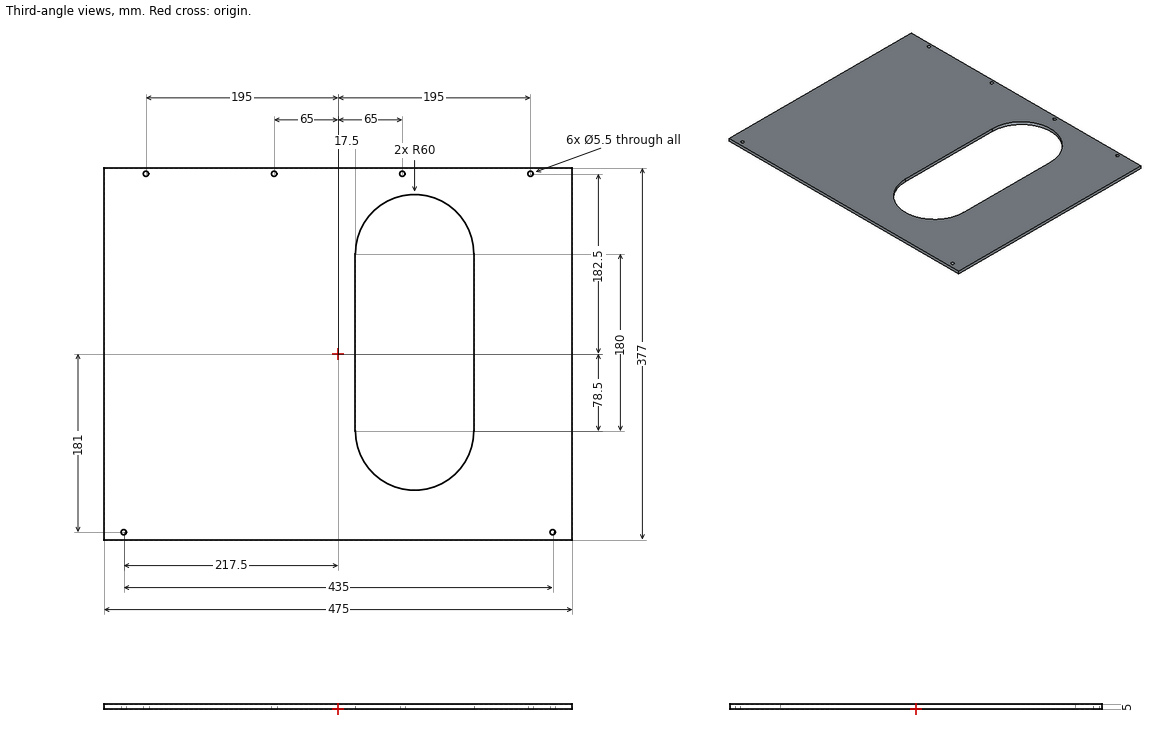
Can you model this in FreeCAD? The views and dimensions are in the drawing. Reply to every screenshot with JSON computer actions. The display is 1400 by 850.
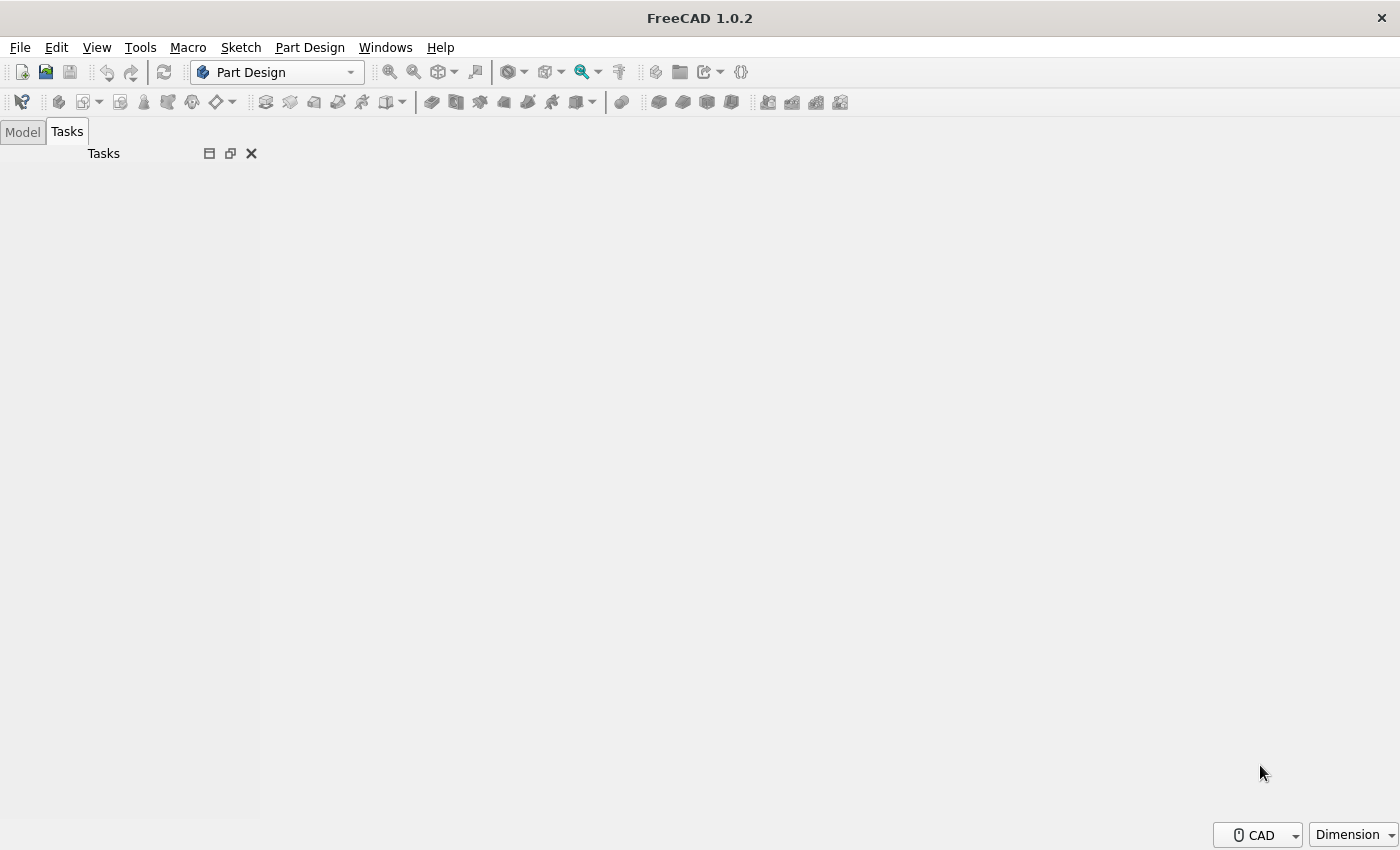
{"action": "key", "text": "ctrl+n"}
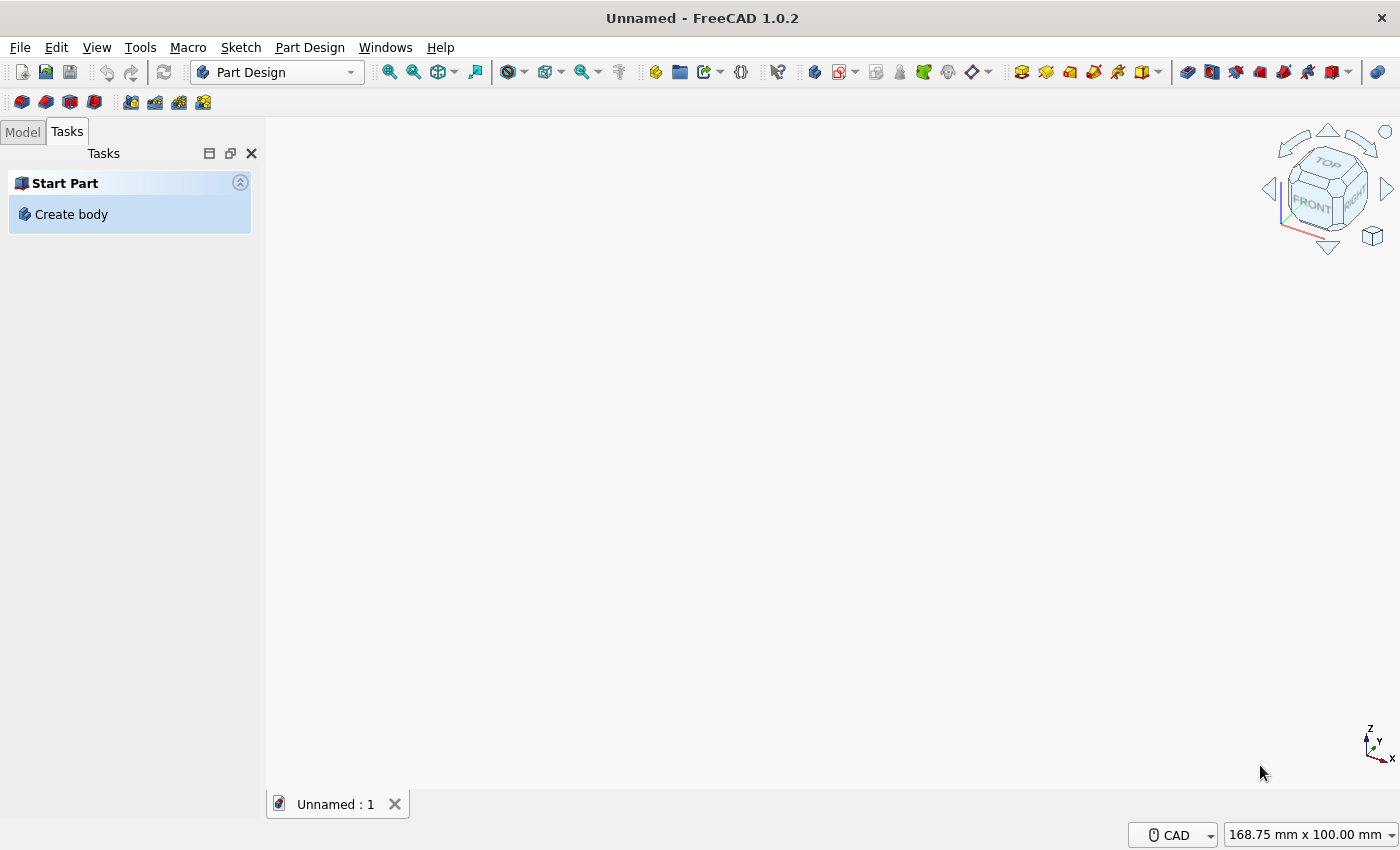
{"action": "left_click", "coordinate": [840, 72]}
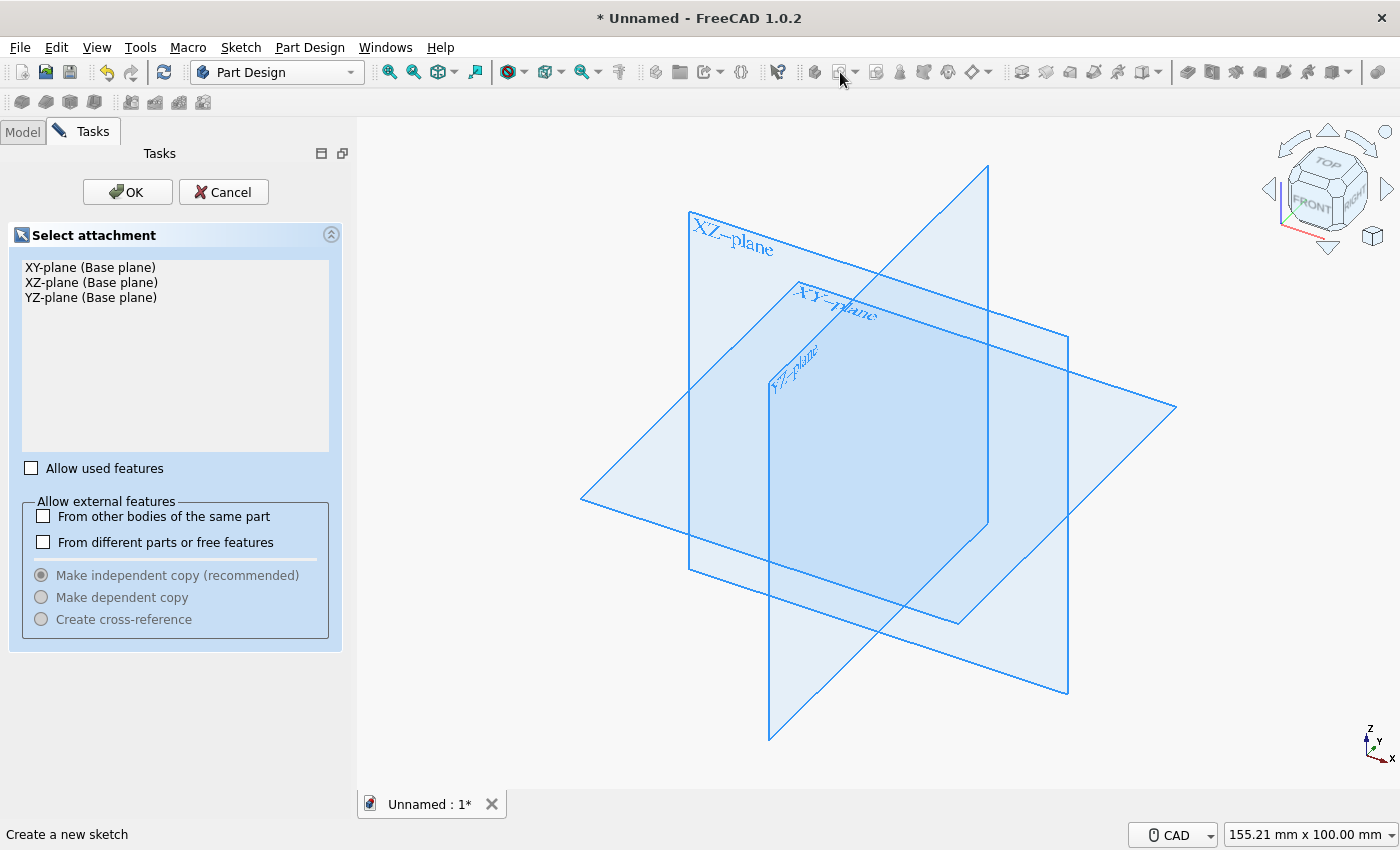
{"action": "left_click", "coordinate": [82, 268]}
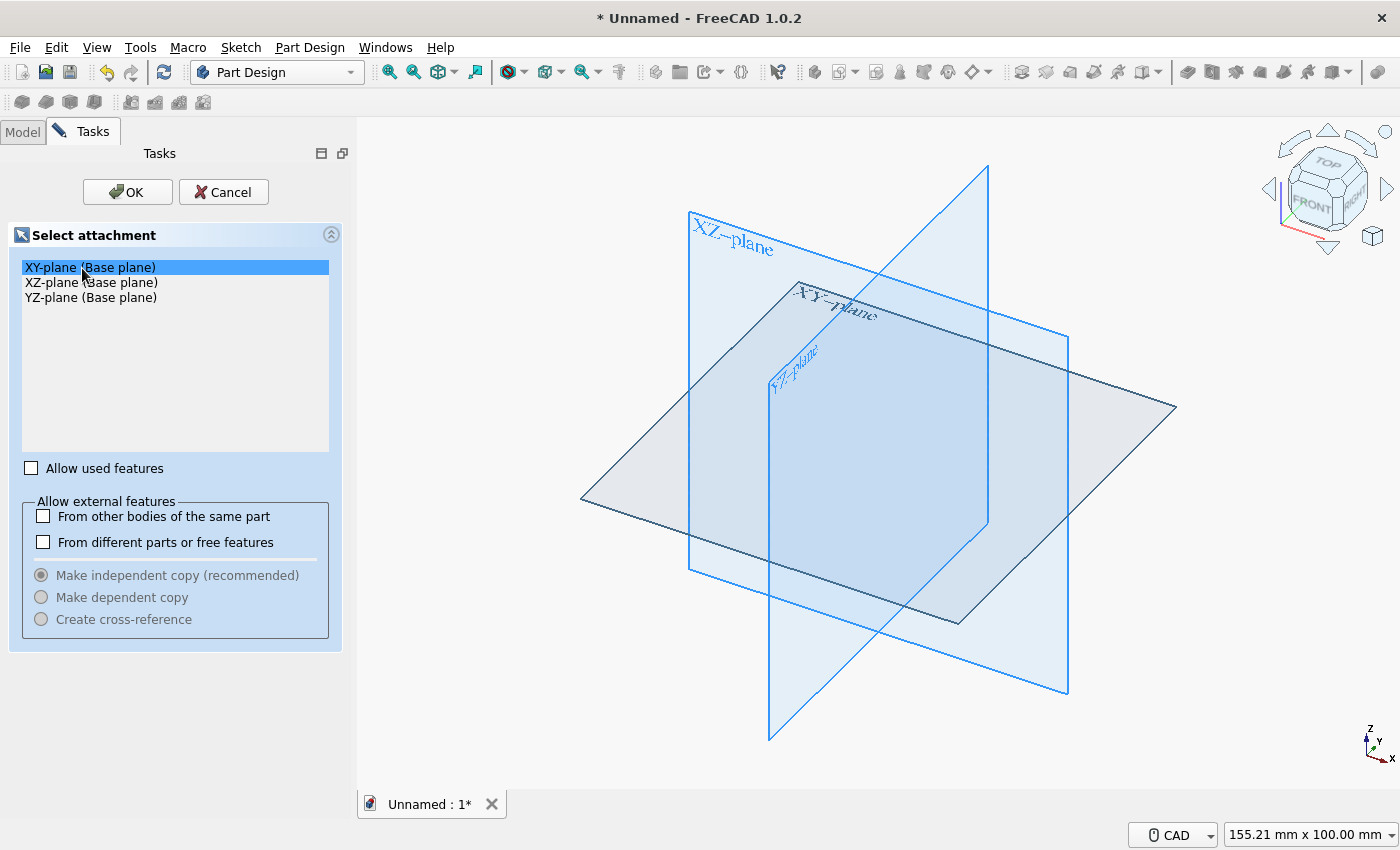
{"action": "left_click", "coordinate": [128, 192]}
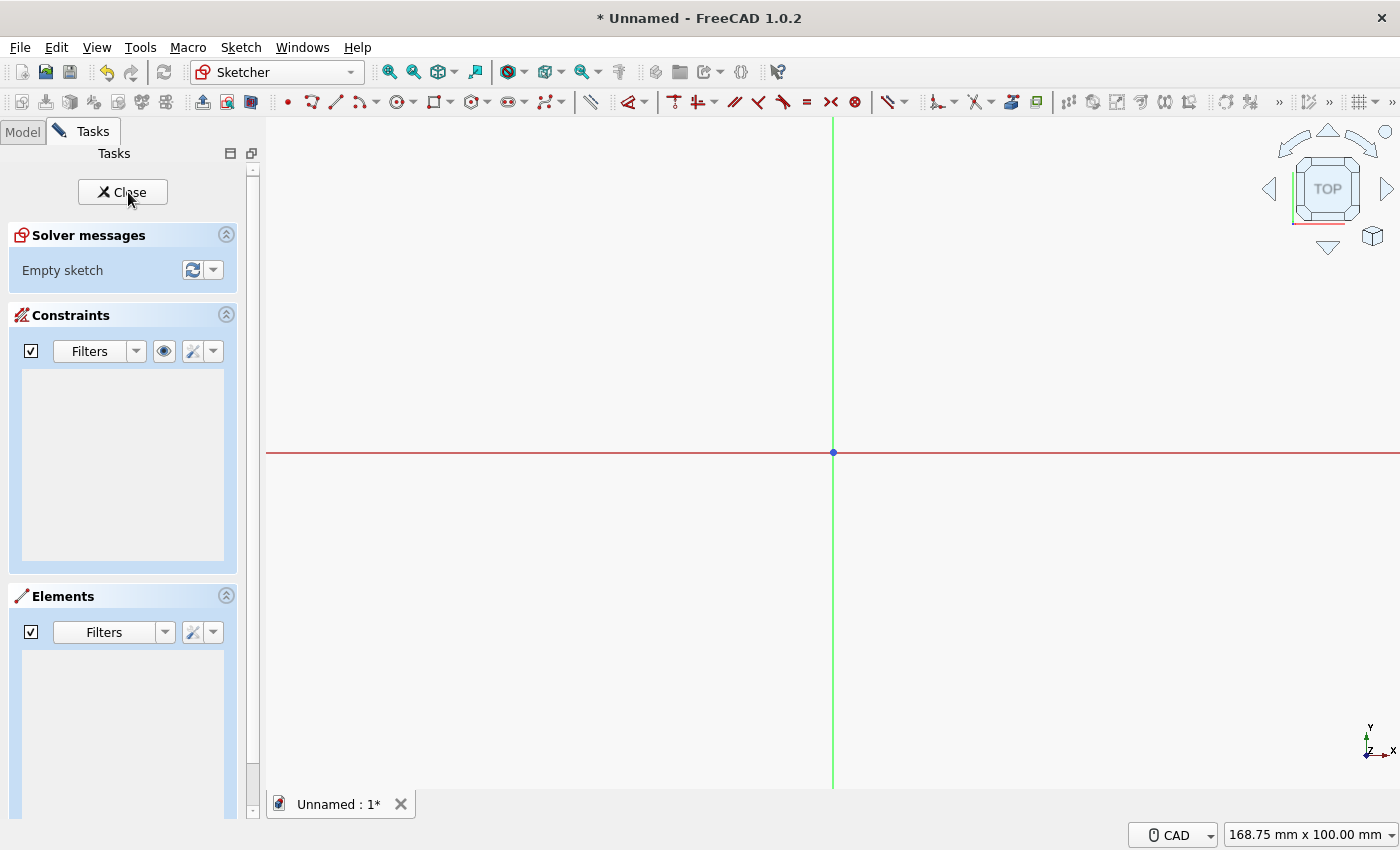
{"action": "scroll", "coordinate": [751, 453], "scroll_direction": "down", "scroll_amount": 9}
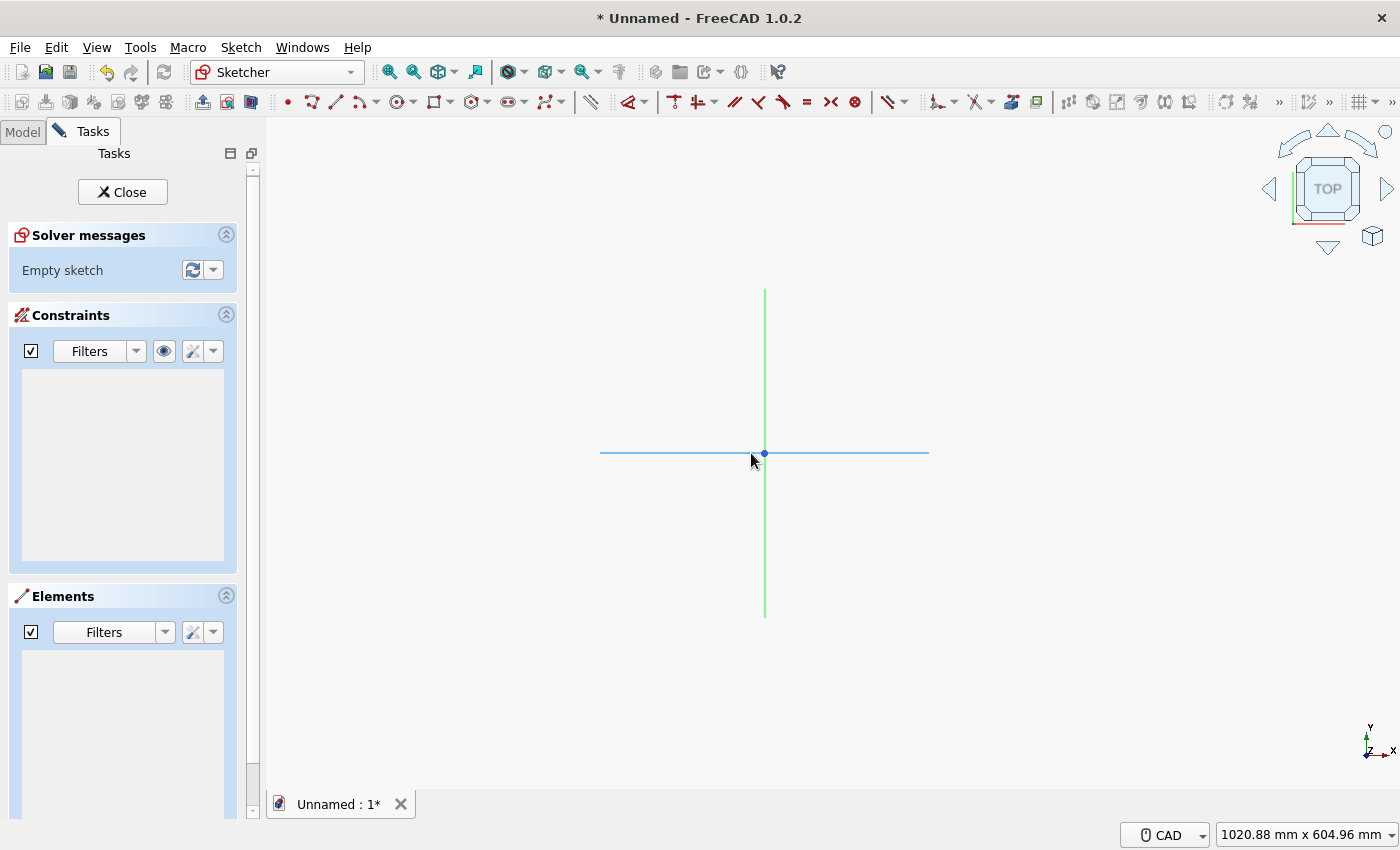
{"action": "left_click", "coordinate": [452, 102]}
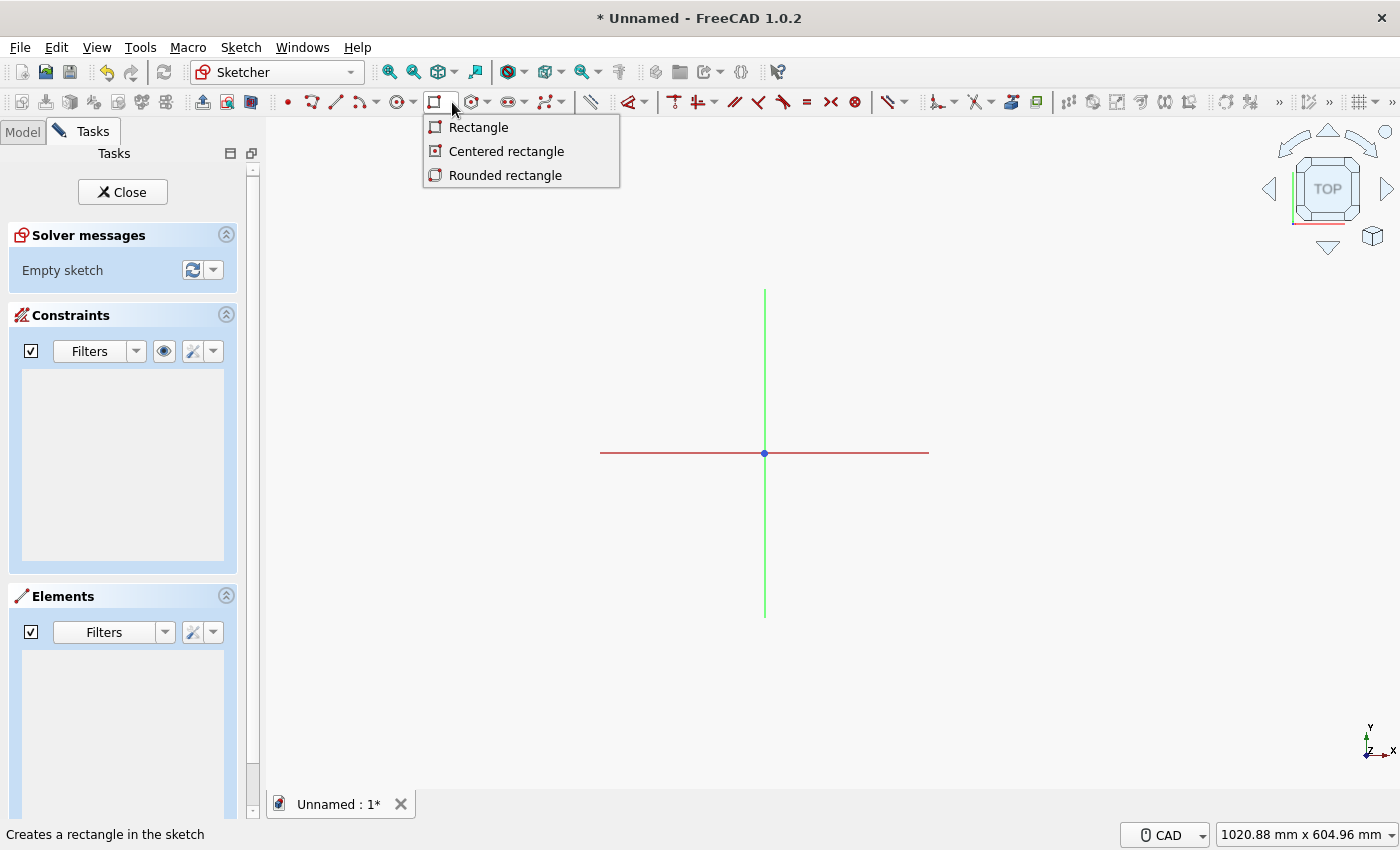
{"action": "left_click", "coordinate": [522, 151]}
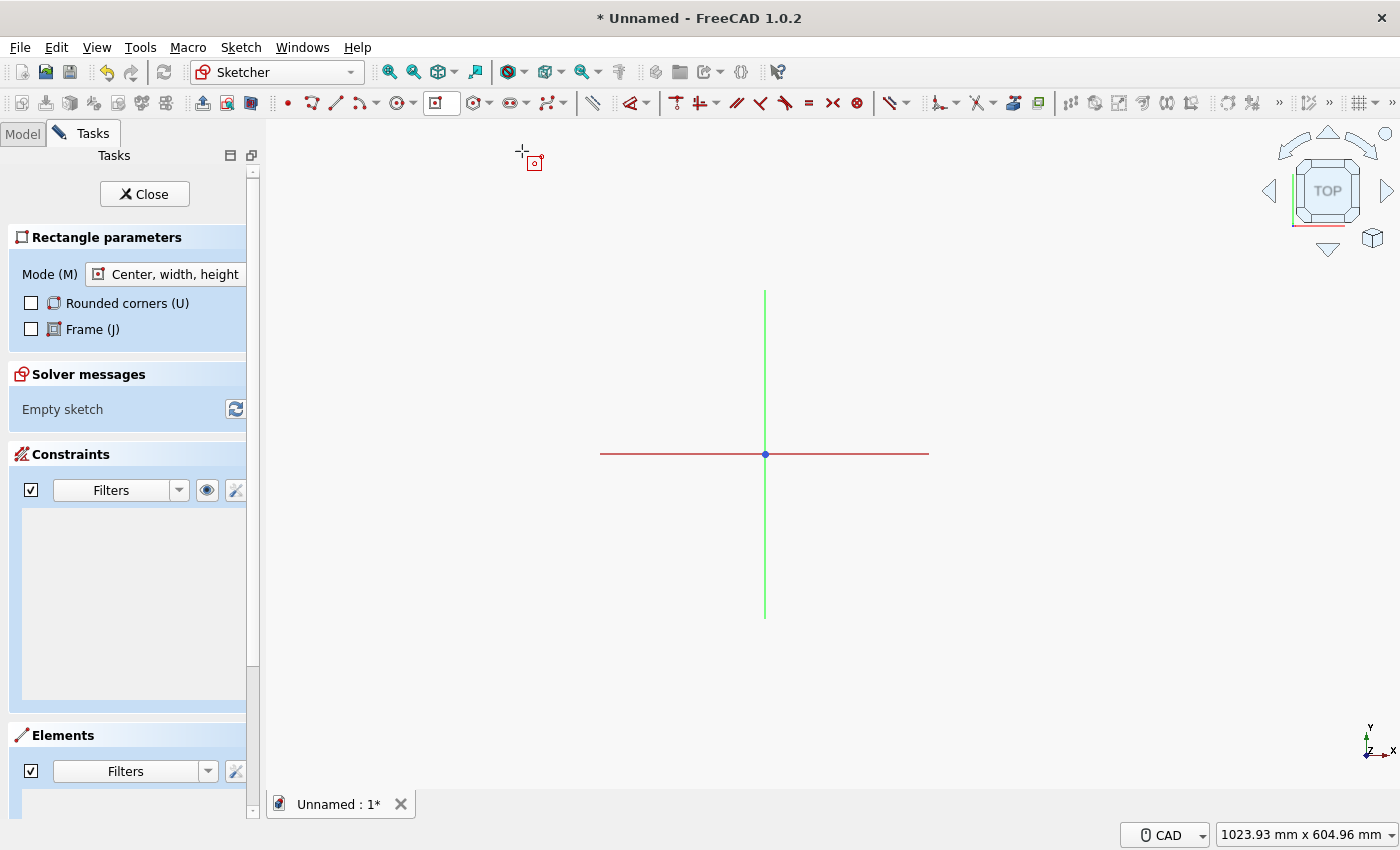
{"action": "left_click", "coordinate": [765, 454]}
{"action": "left_click", "coordinate": [1028, 246]}
{"action": "key", "text": "Escape"}